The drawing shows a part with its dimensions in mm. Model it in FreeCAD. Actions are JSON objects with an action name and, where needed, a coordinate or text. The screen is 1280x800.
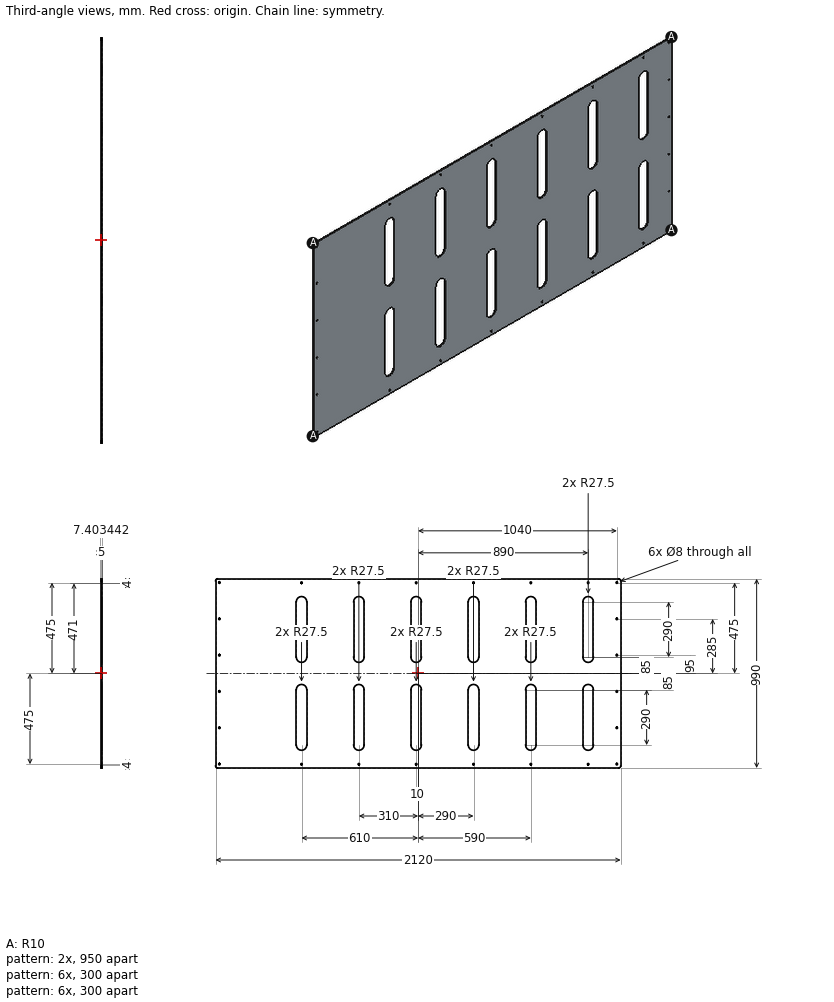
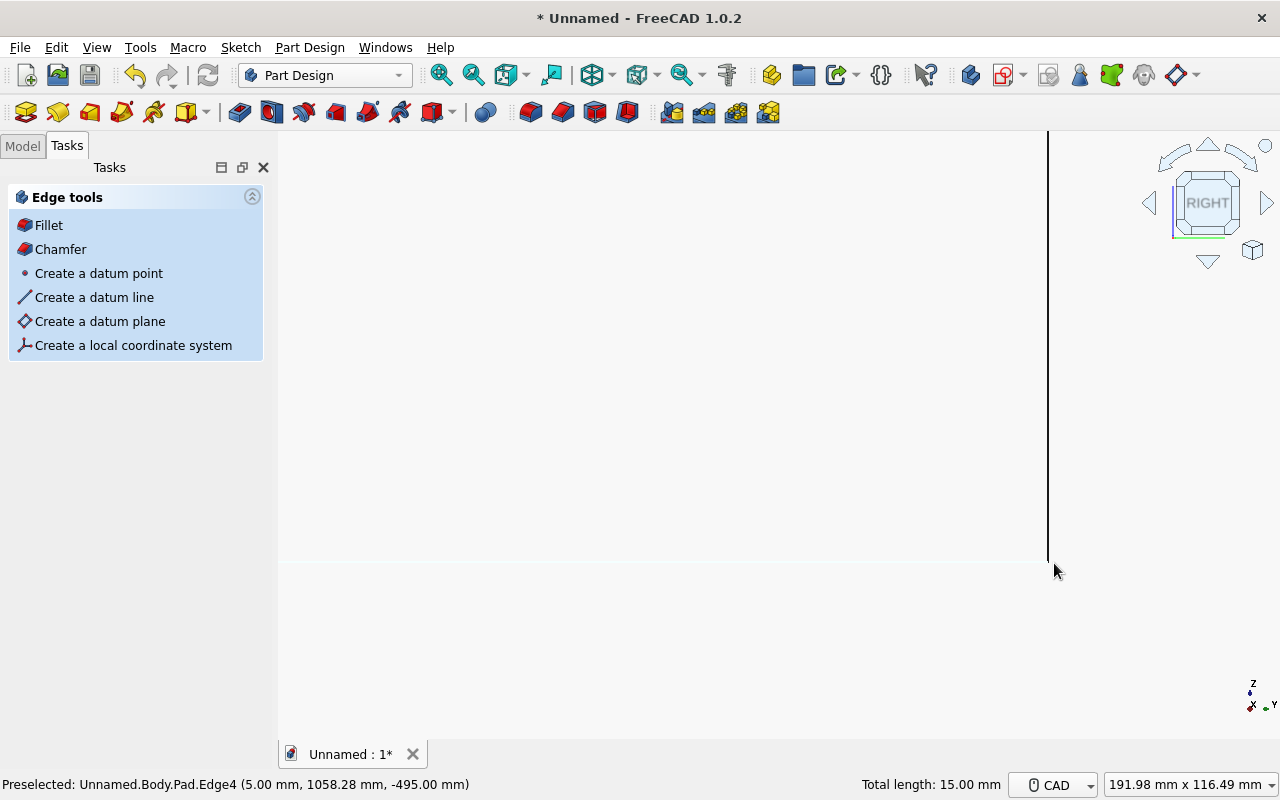
{"action": "left_click", "coordinate": [442, 76]}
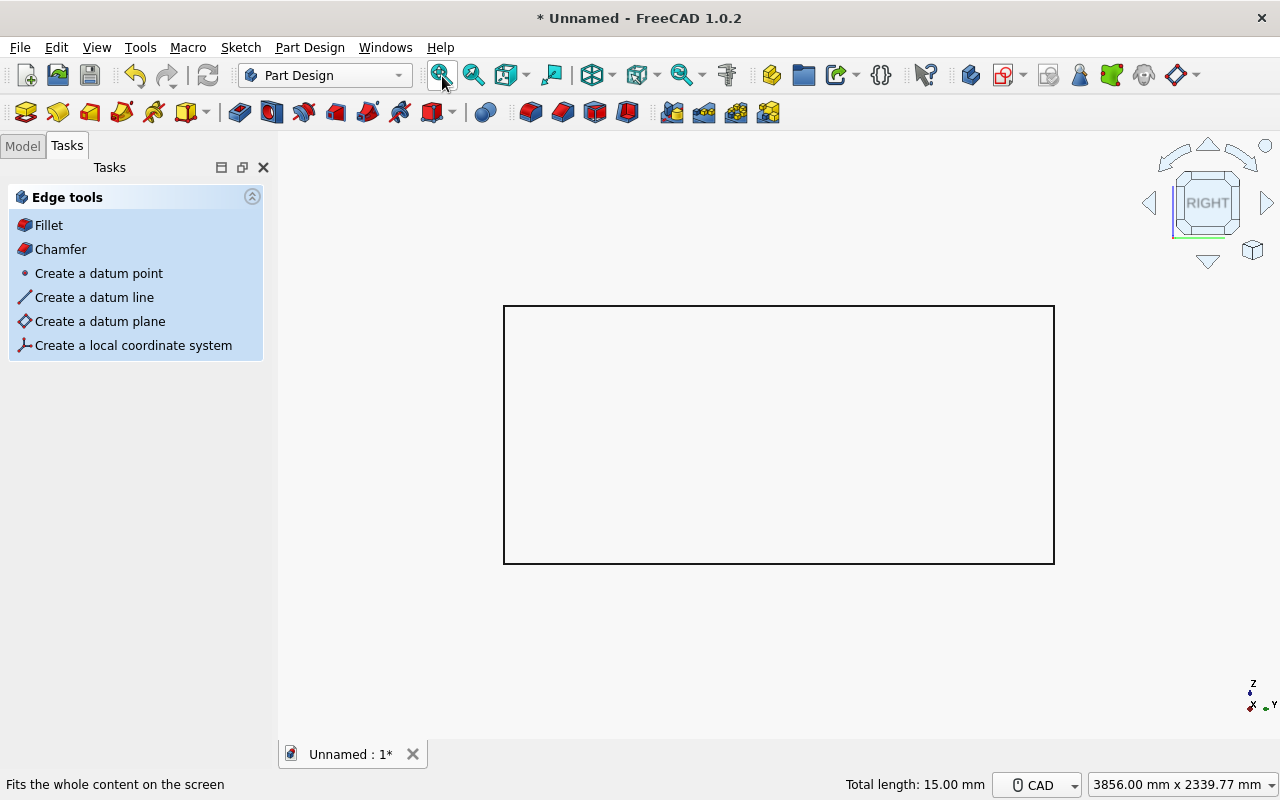
{"action": "key", "text": "5"}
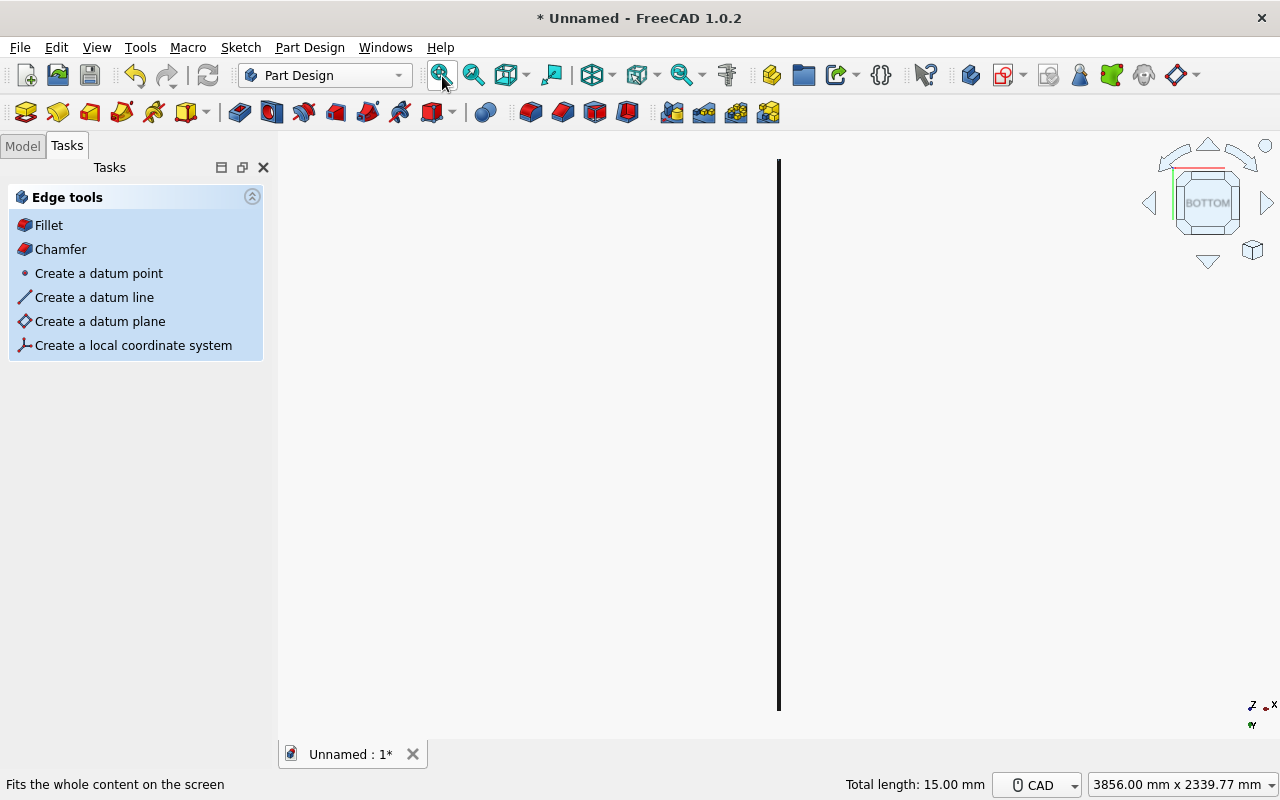
{"action": "left_click", "coordinate": [779, 709], "text": "ctrl"}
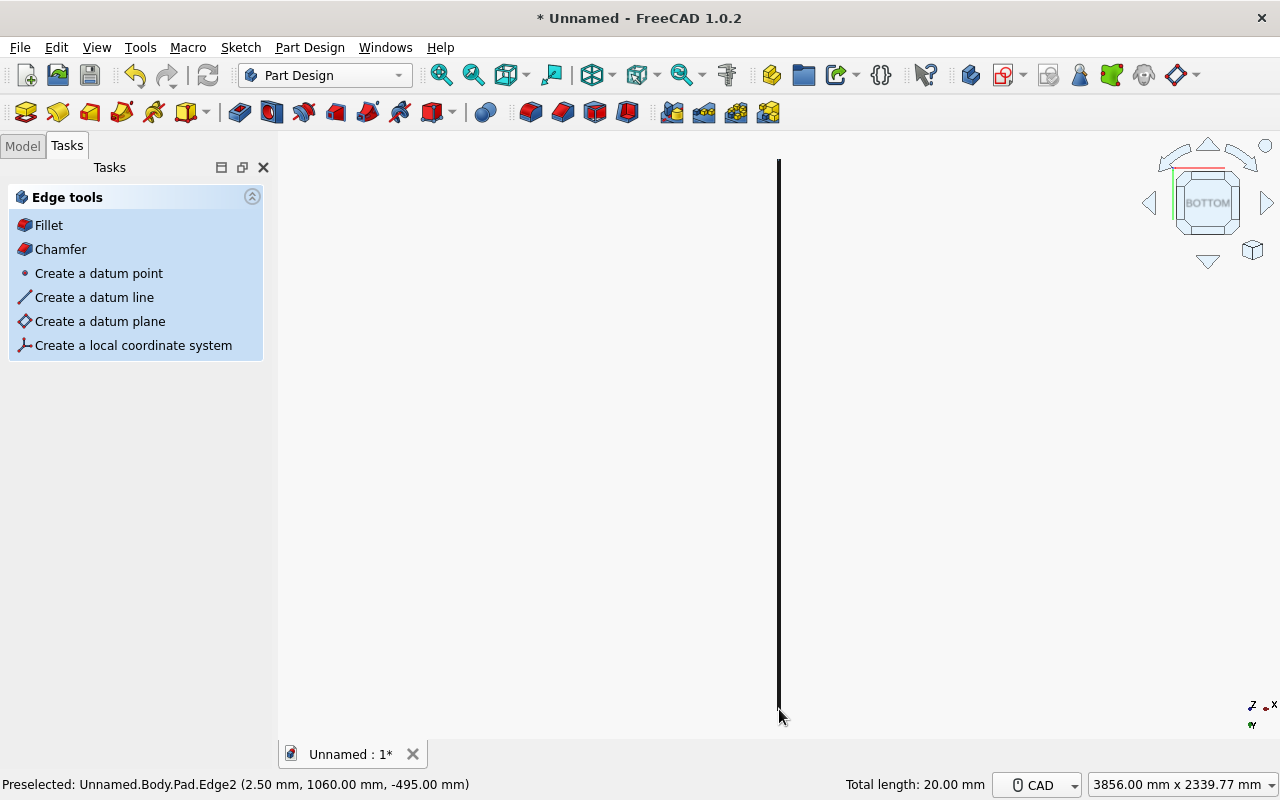
{"action": "key", "text": "v 1"}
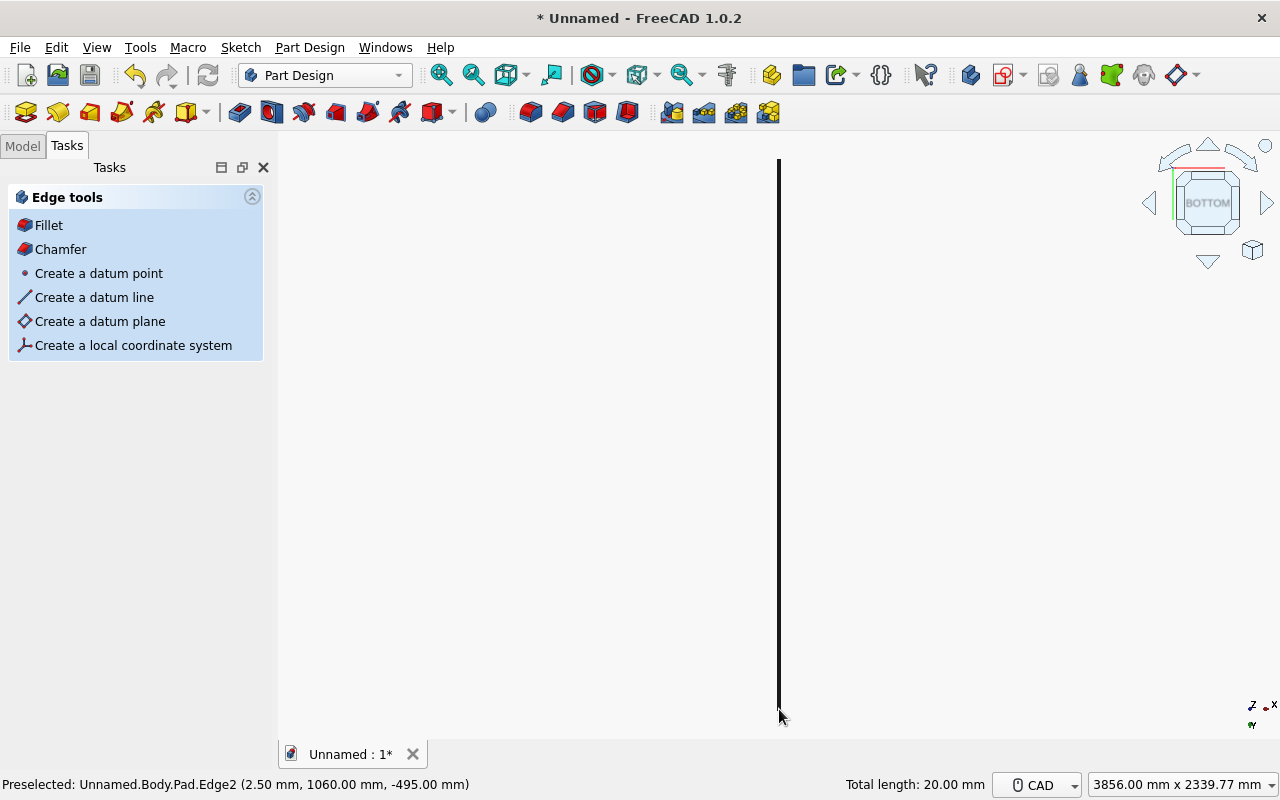
{"action": "left_click", "coordinate": [532, 112]}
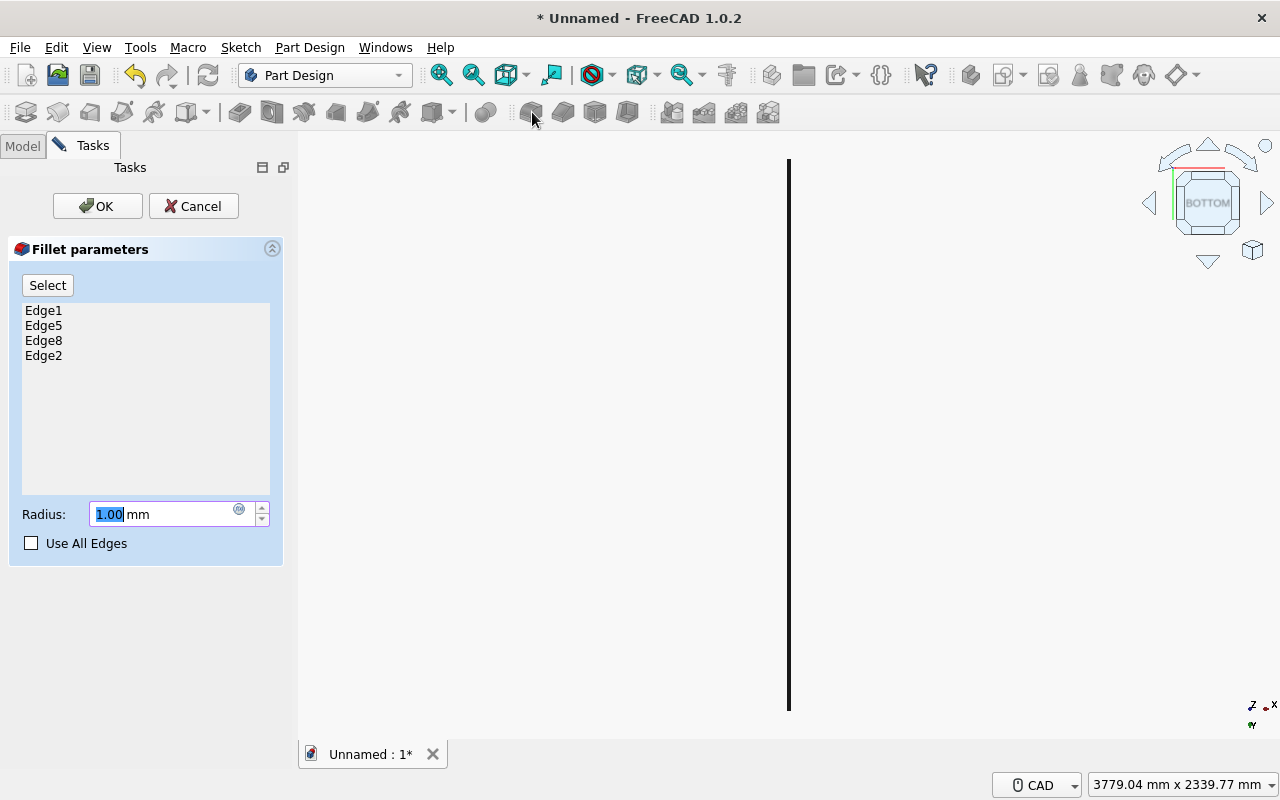
{"action": "type", "text": "10"}
{"action": "key", "text": "Tab"}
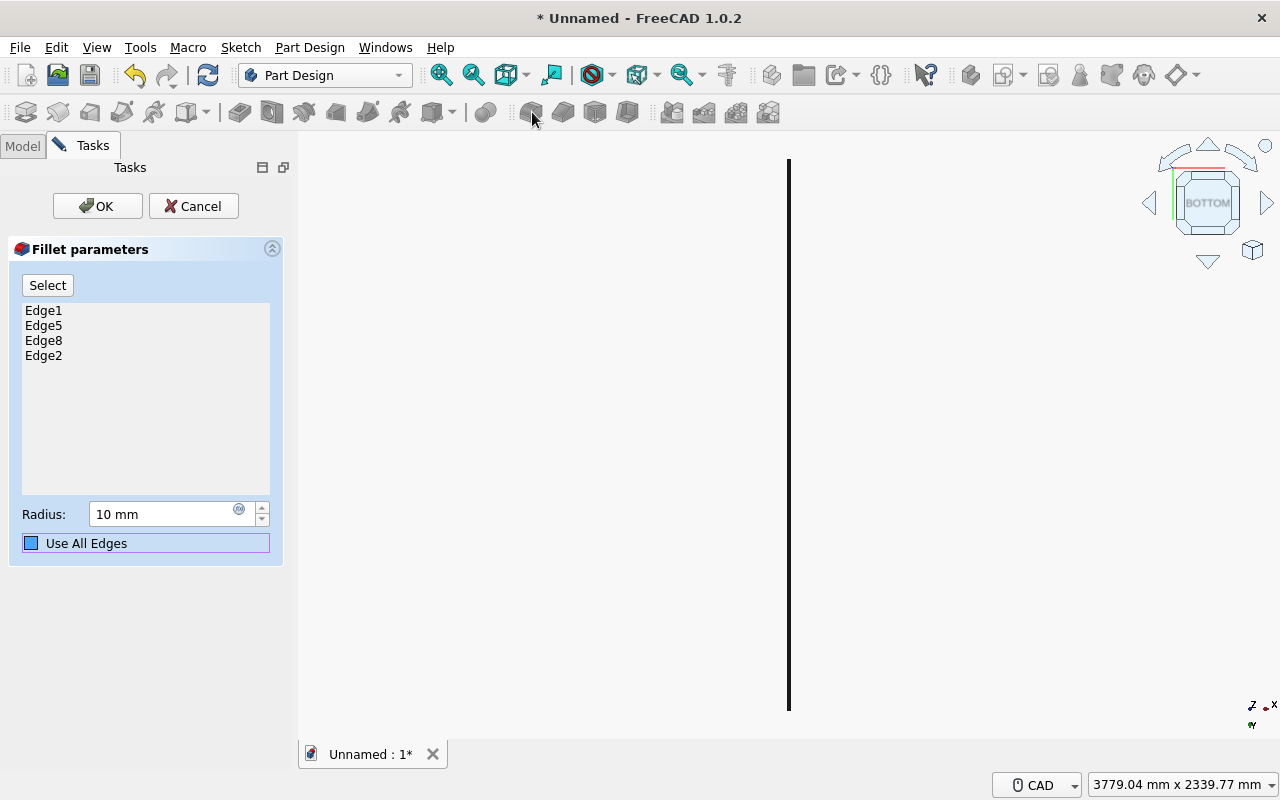
{"action": "left_click", "coordinate": [98, 206]}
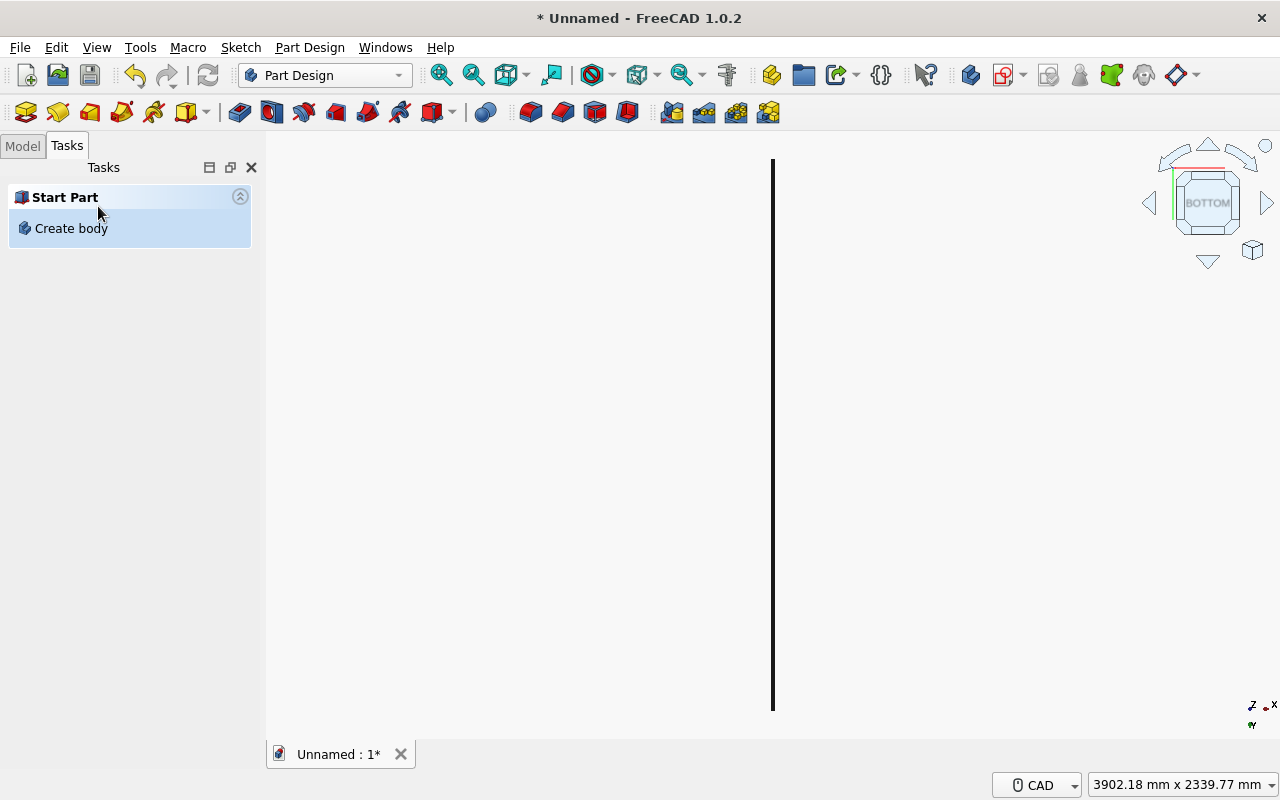
{"action": "key", "text": "0"}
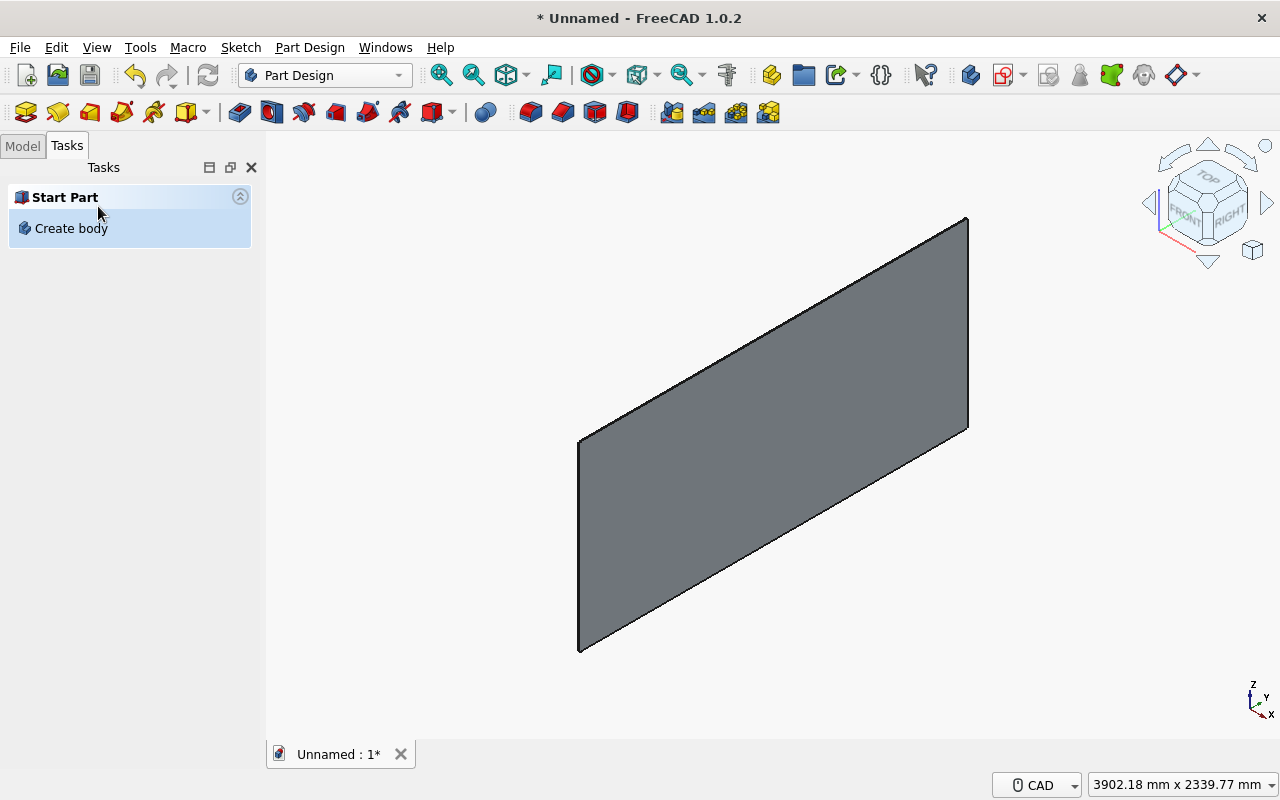
{"action": "left_click", "coordinate": [829, 402]}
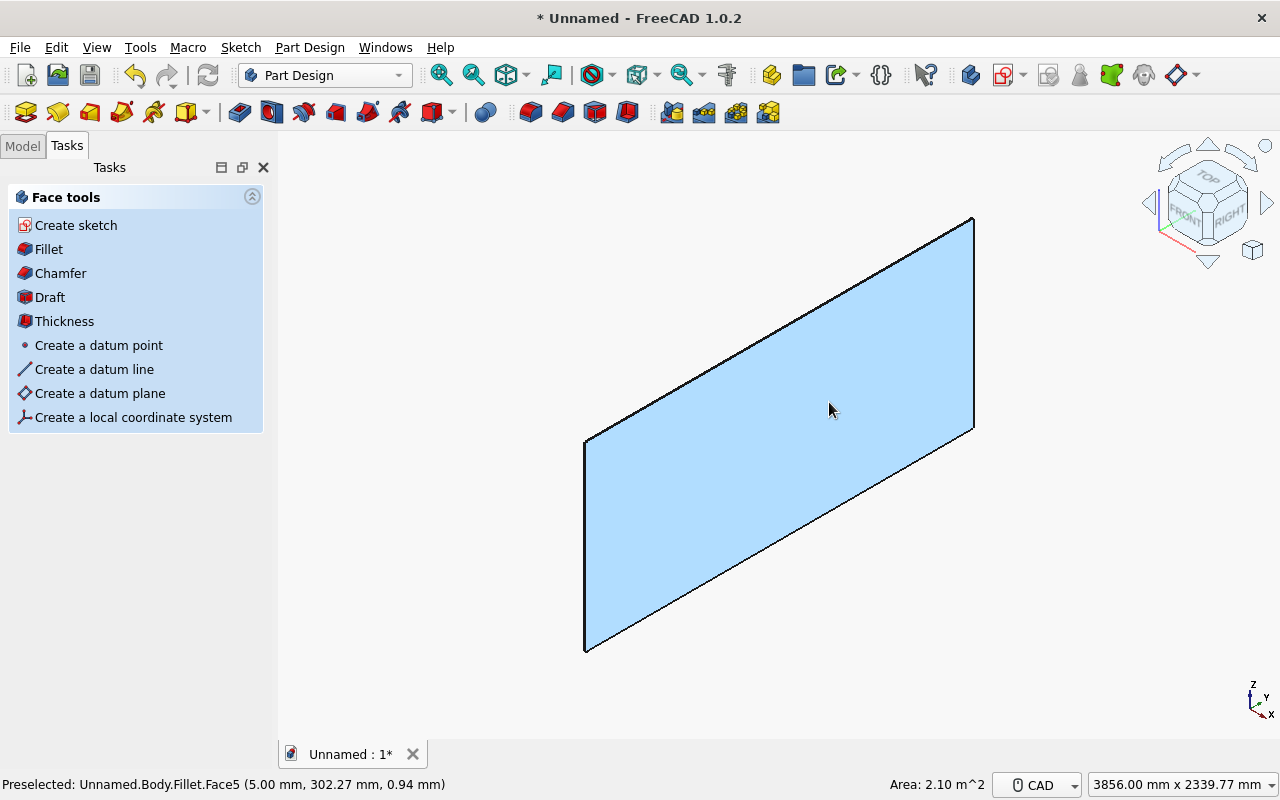
{"action": "left_click", "coordinate": [1004, 76]}